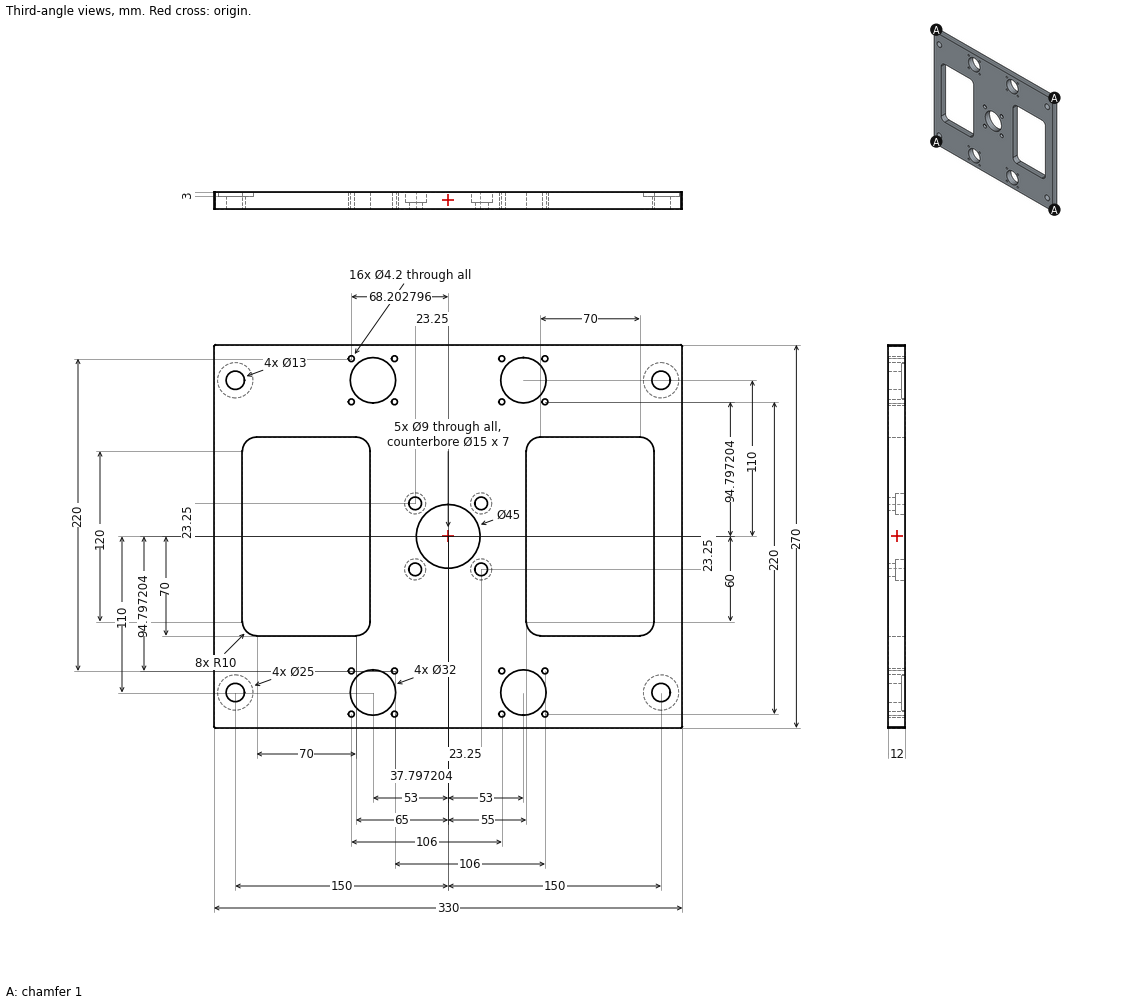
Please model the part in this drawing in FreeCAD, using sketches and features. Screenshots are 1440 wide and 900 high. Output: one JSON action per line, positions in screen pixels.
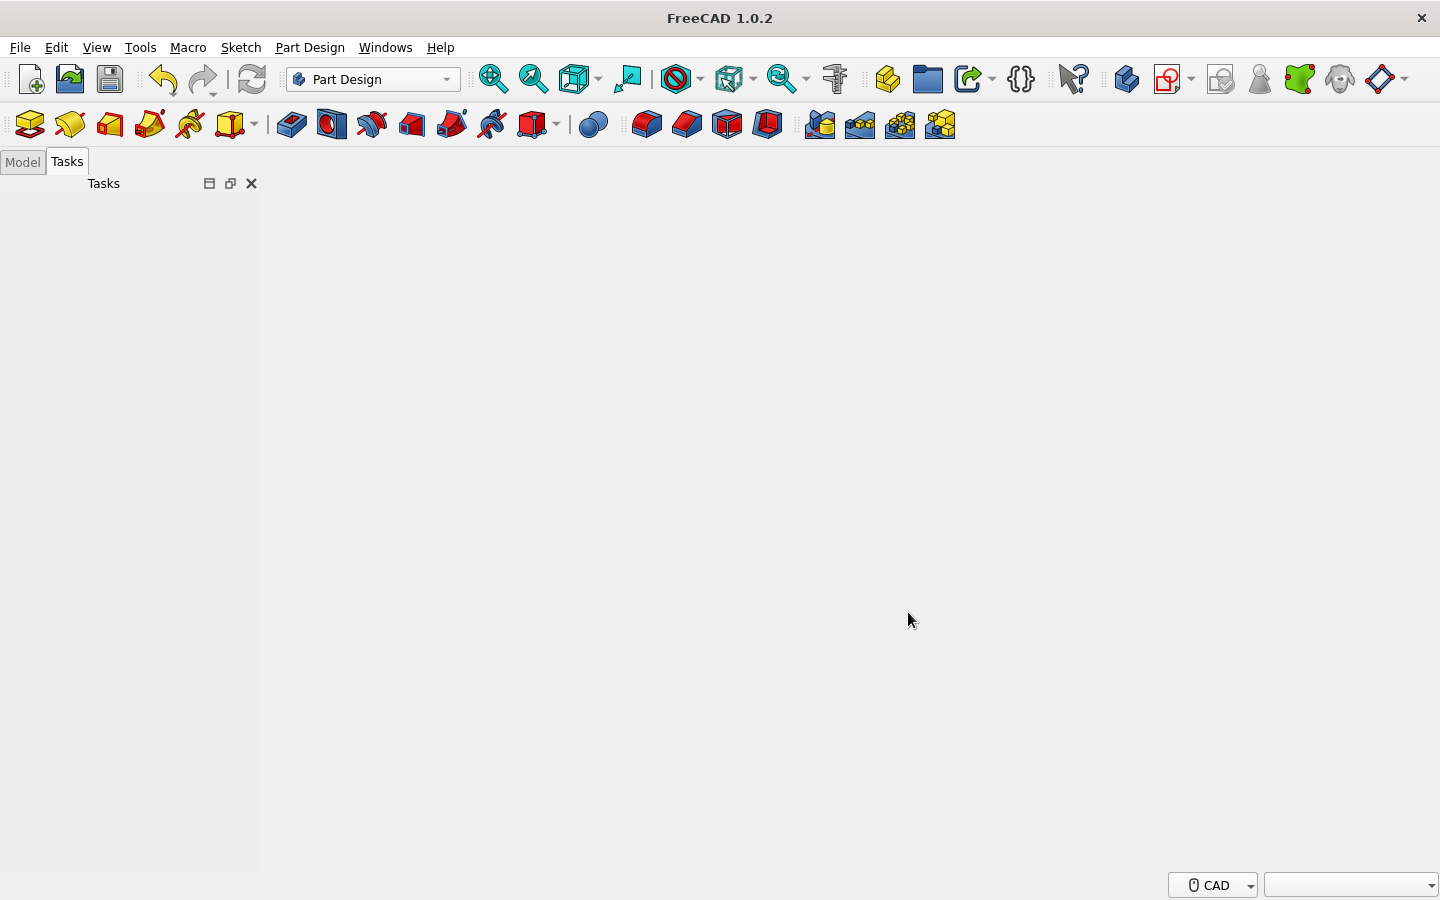
{"action": "left_click", "coordinate": [30, 80]}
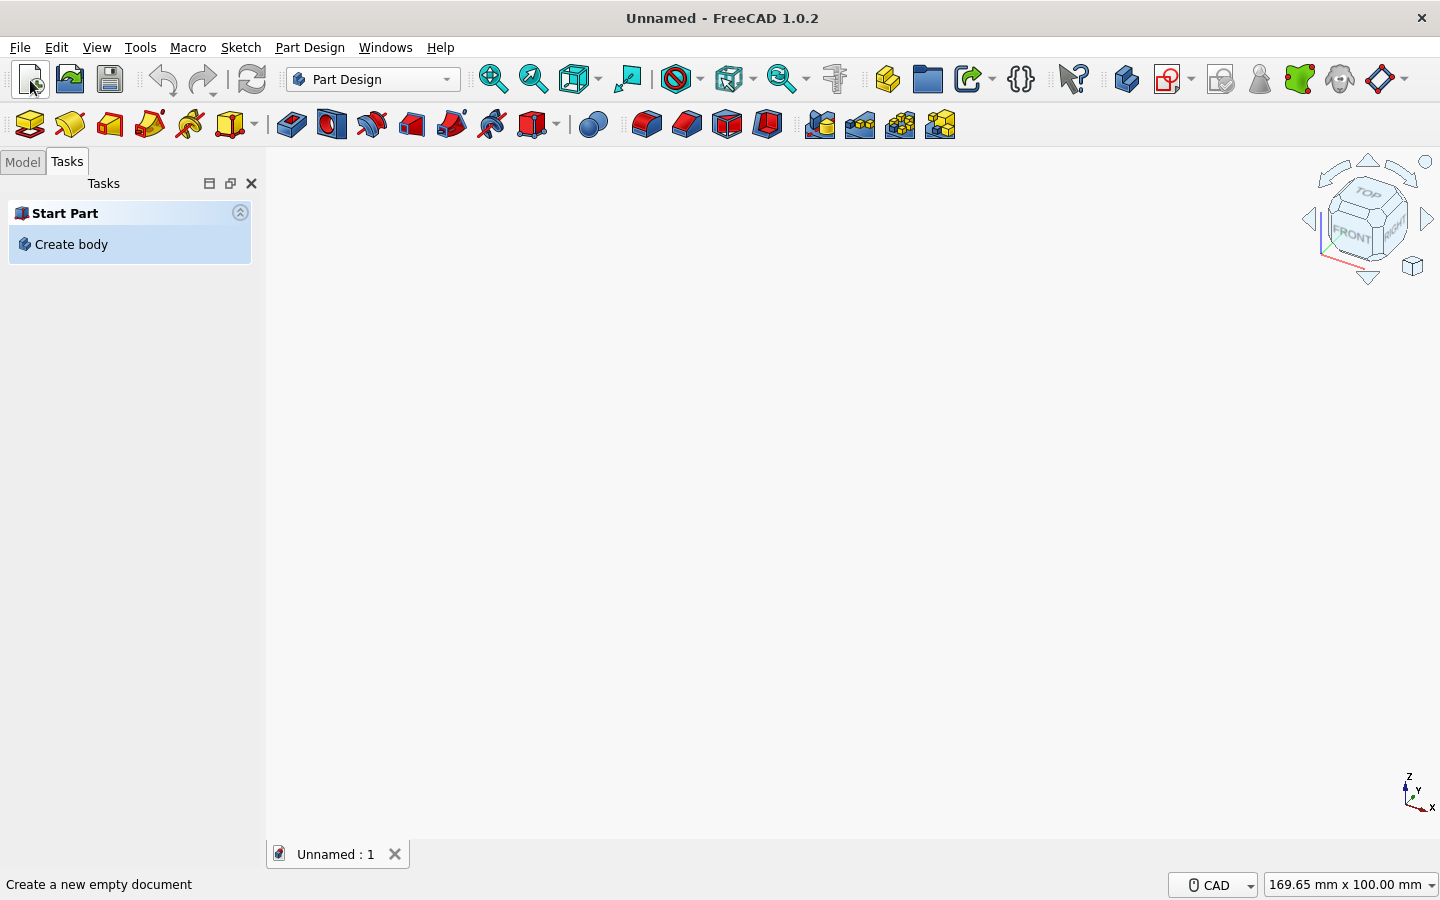
{"action": "left_click", "coordinate": [1168, 80]}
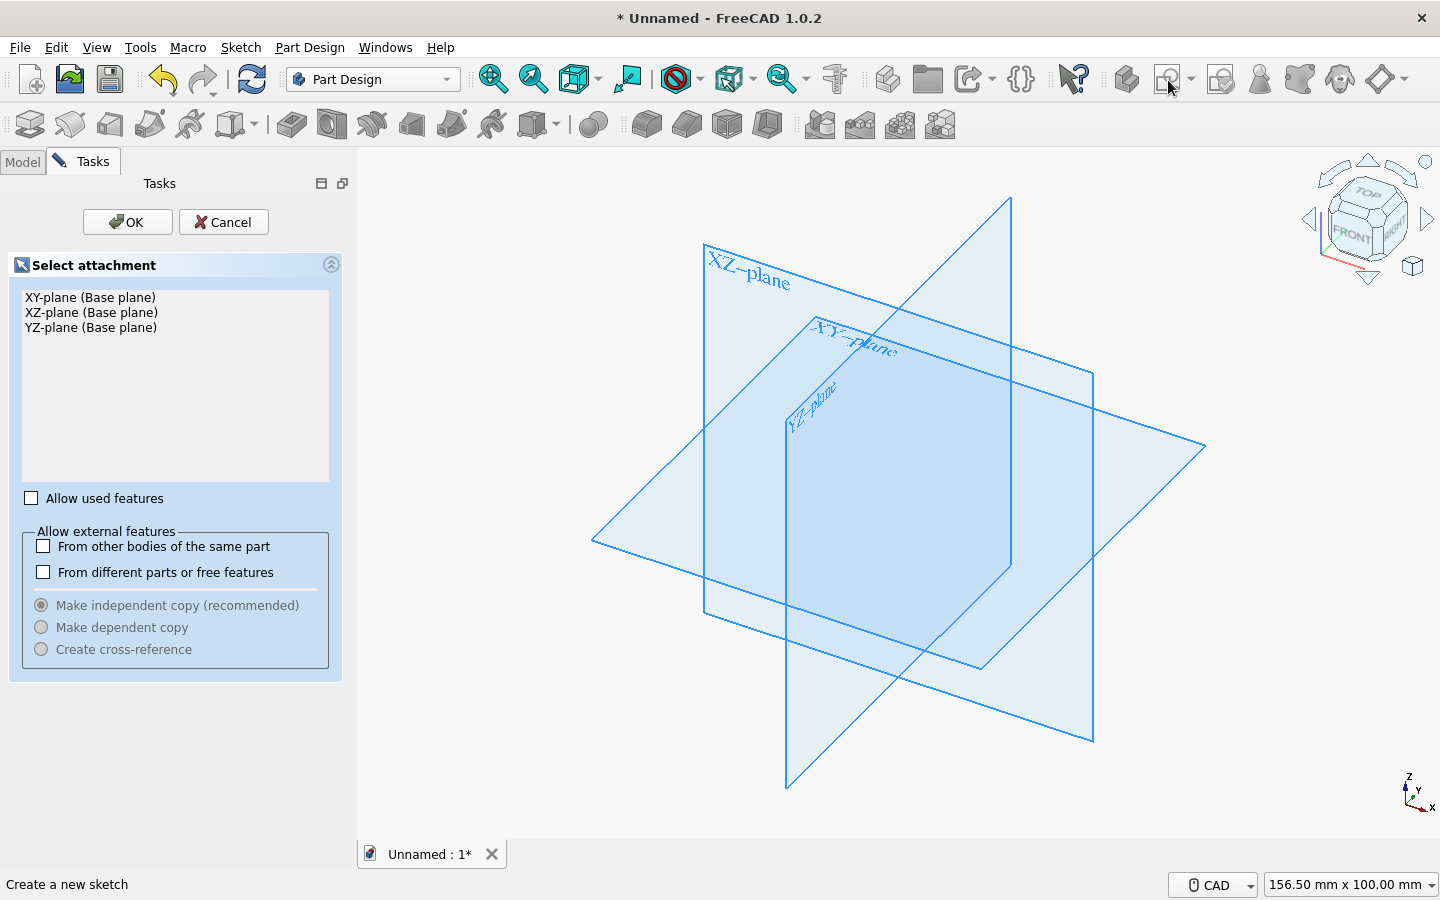
{"action": "left_click", "coordinate": [82, 312]}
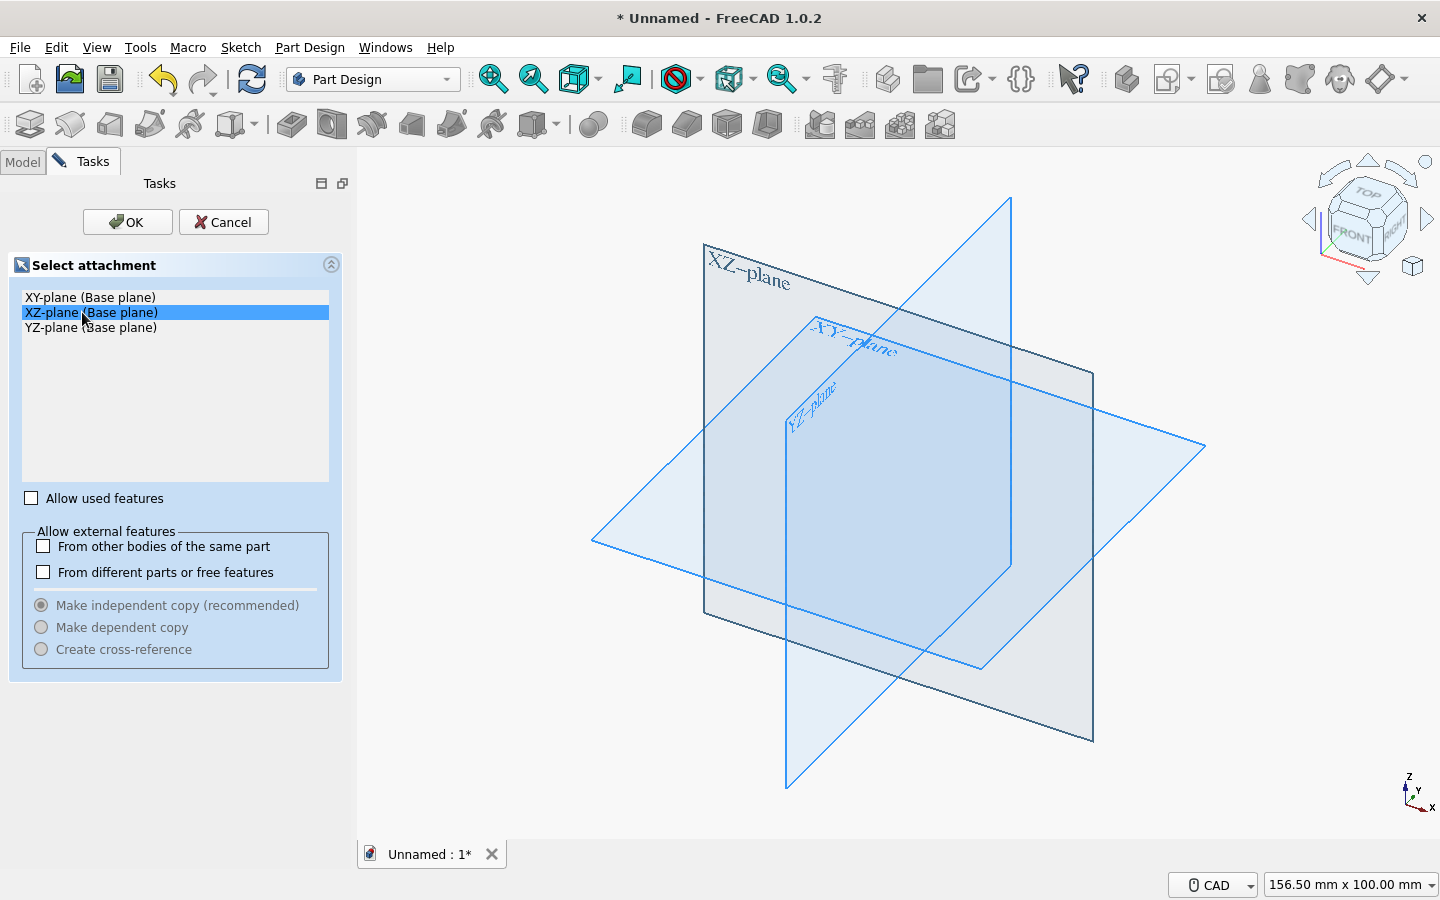
{"action": "left_click", "coordinate": [128, 222]}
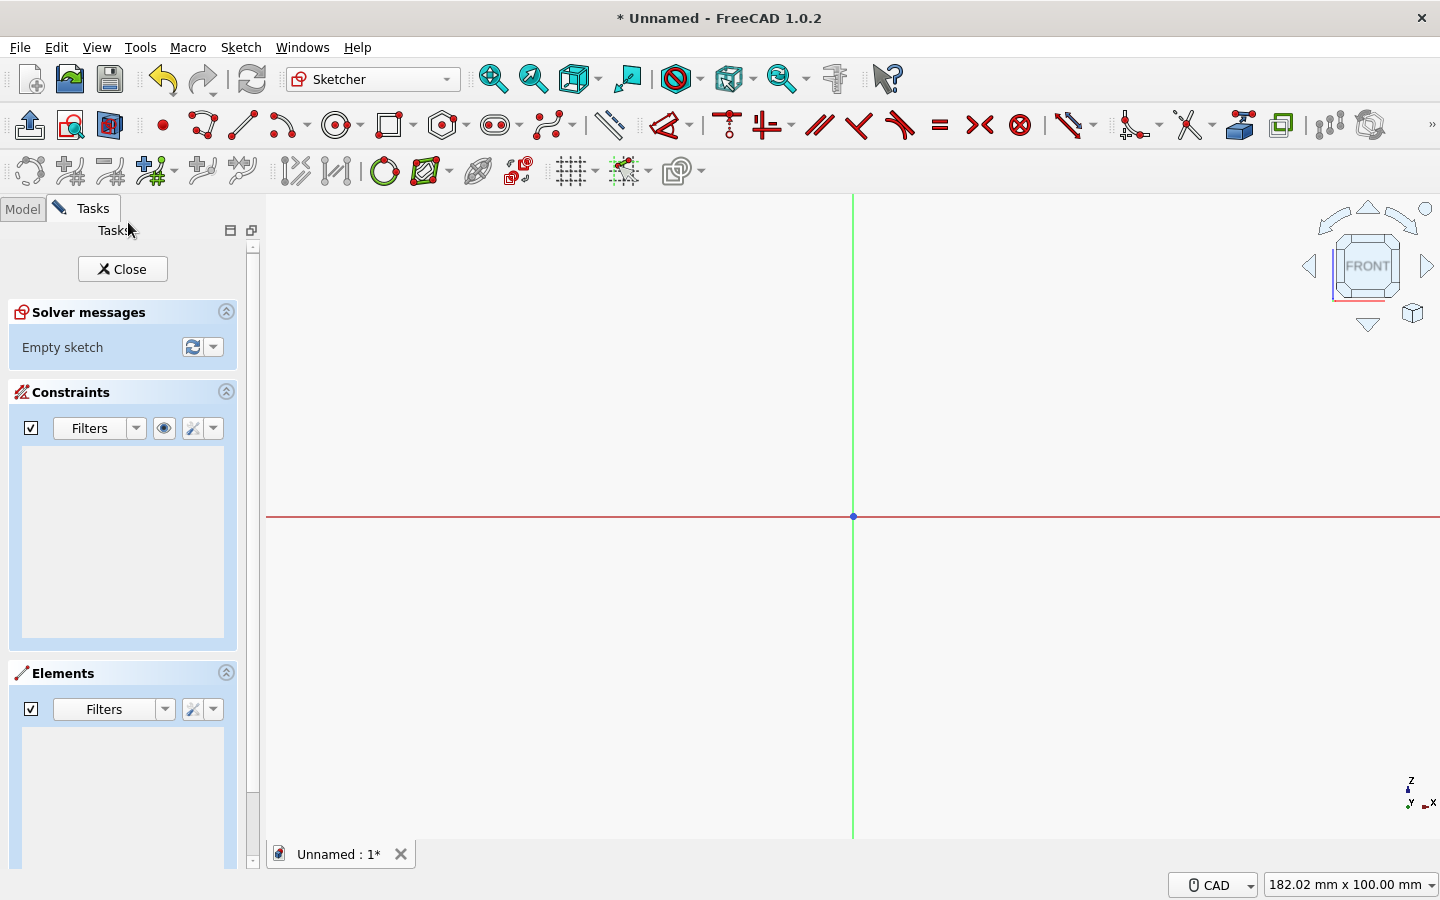
{"action": "scroll", "coordinate": [762, 516], "scroll_direction": "down", "scroll_amount": 7}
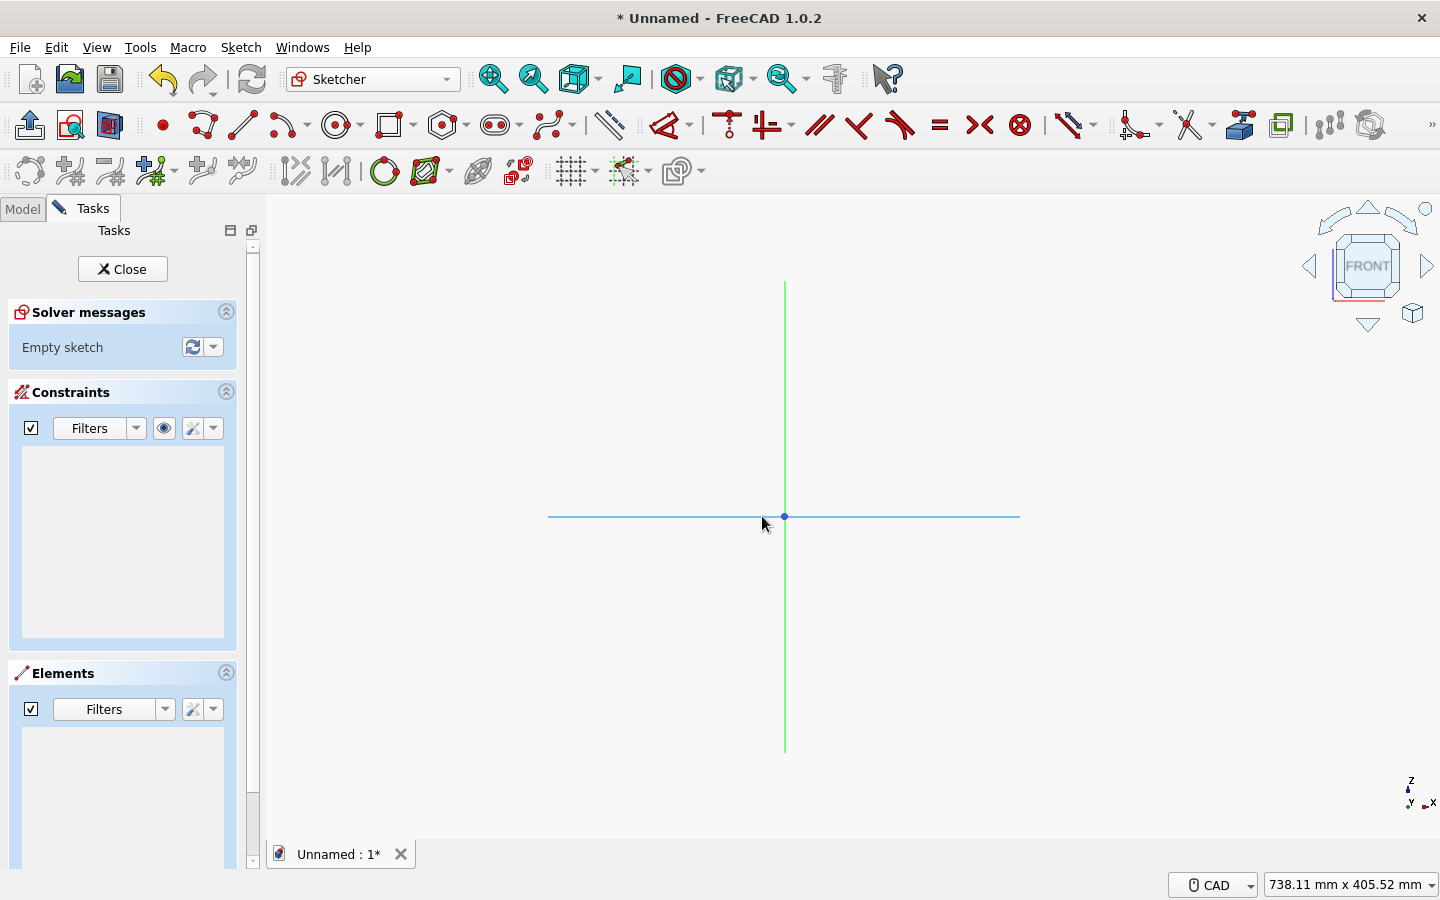
{"action": "key", "text": "g v"}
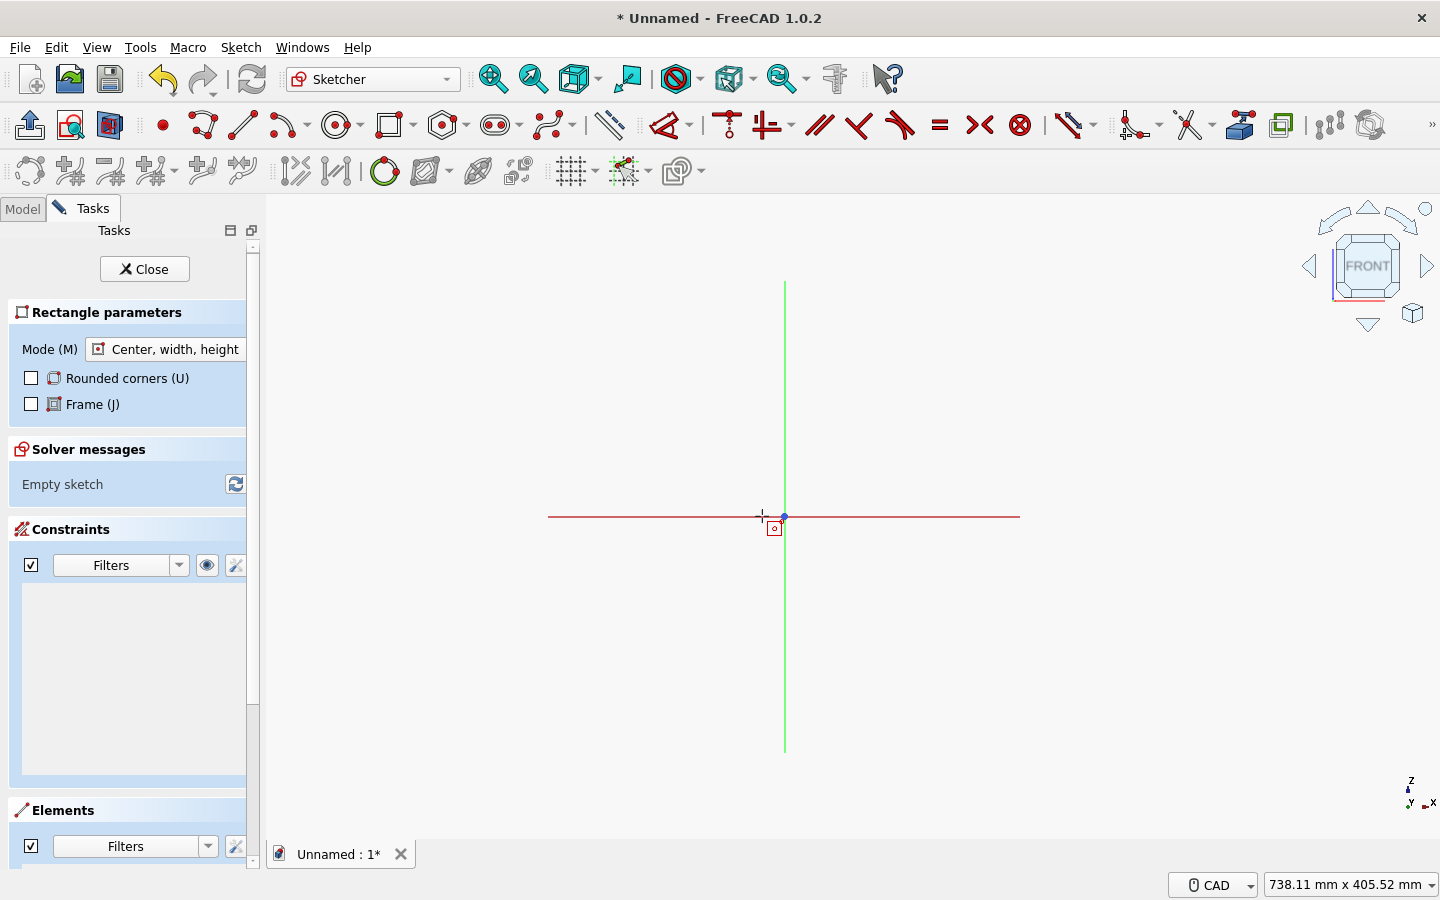
{"action": "left_click", "coordinate": [785, 516]}
{"action": "mouse_move", "coordinate": [1047, 302]}